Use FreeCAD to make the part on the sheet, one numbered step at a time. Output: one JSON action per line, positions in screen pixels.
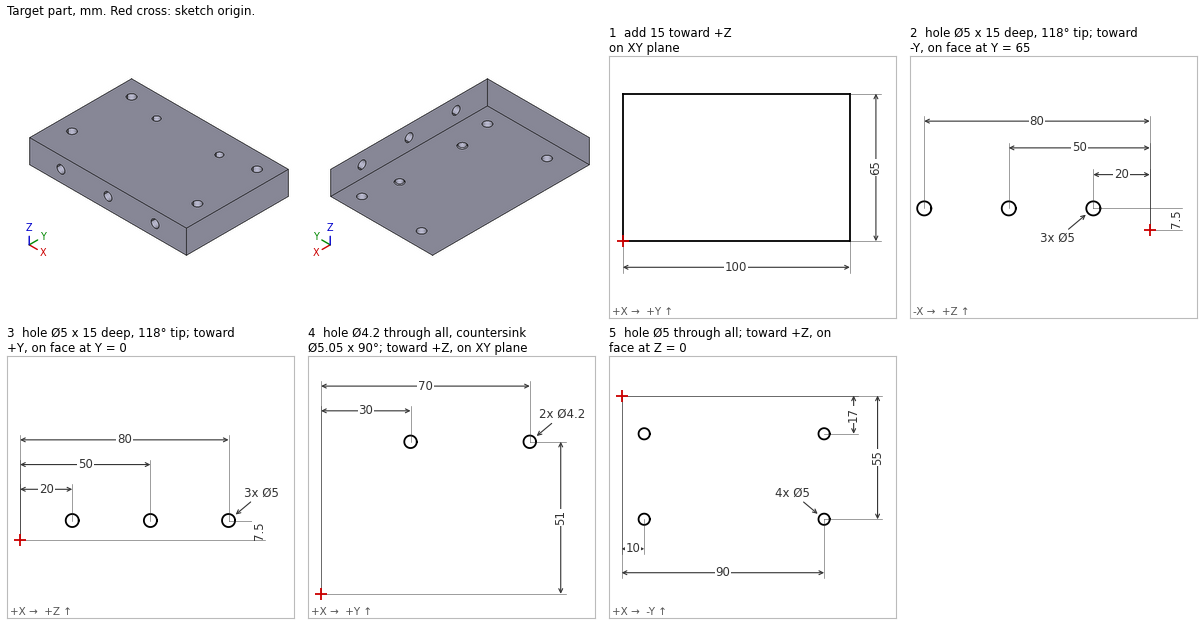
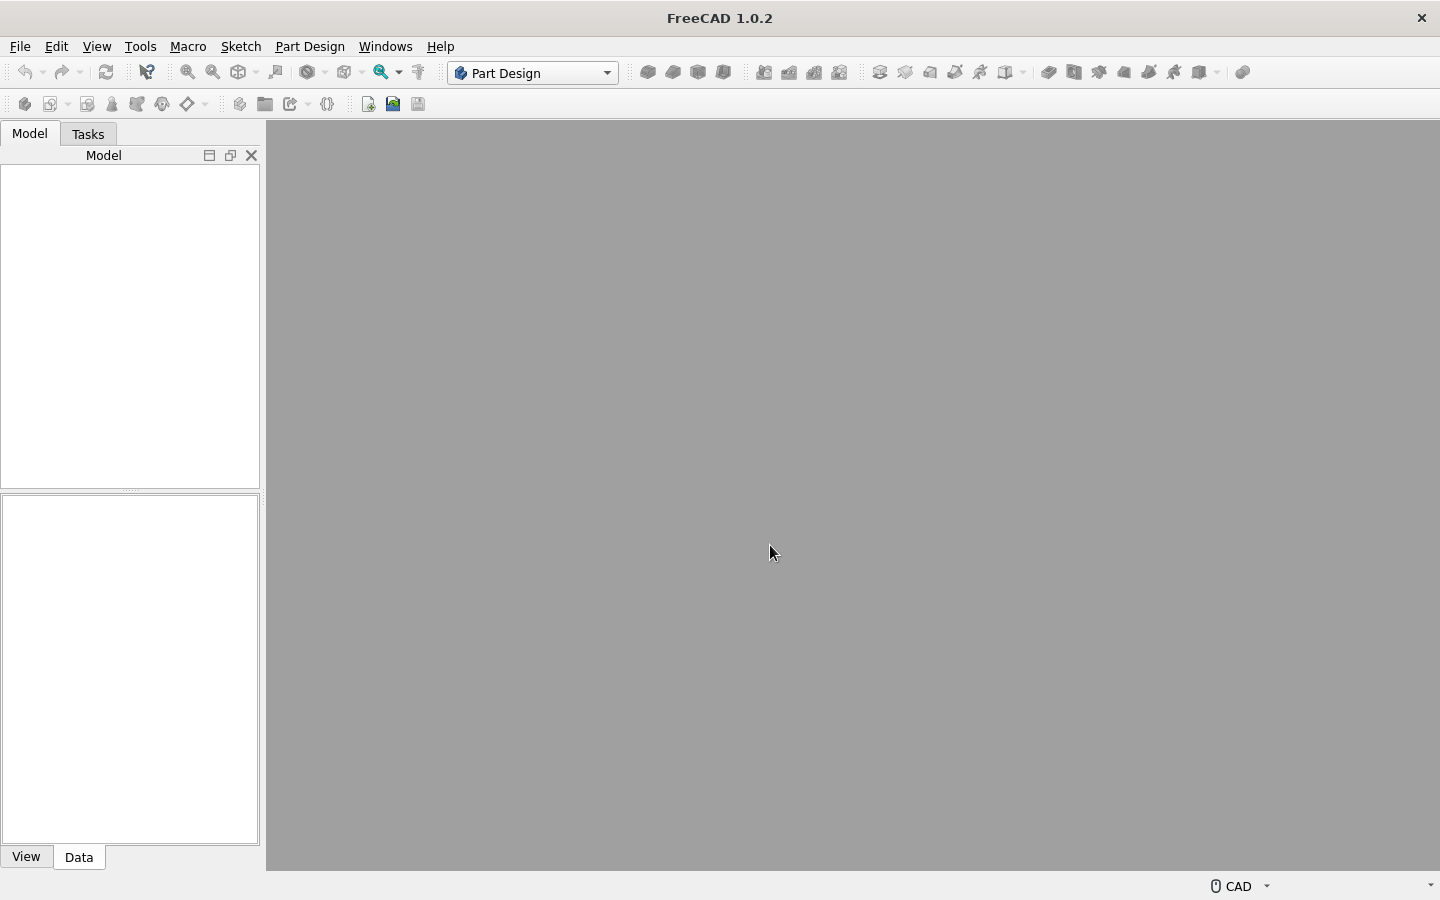
{"action": "left_click", "coordinate": [368, 104]}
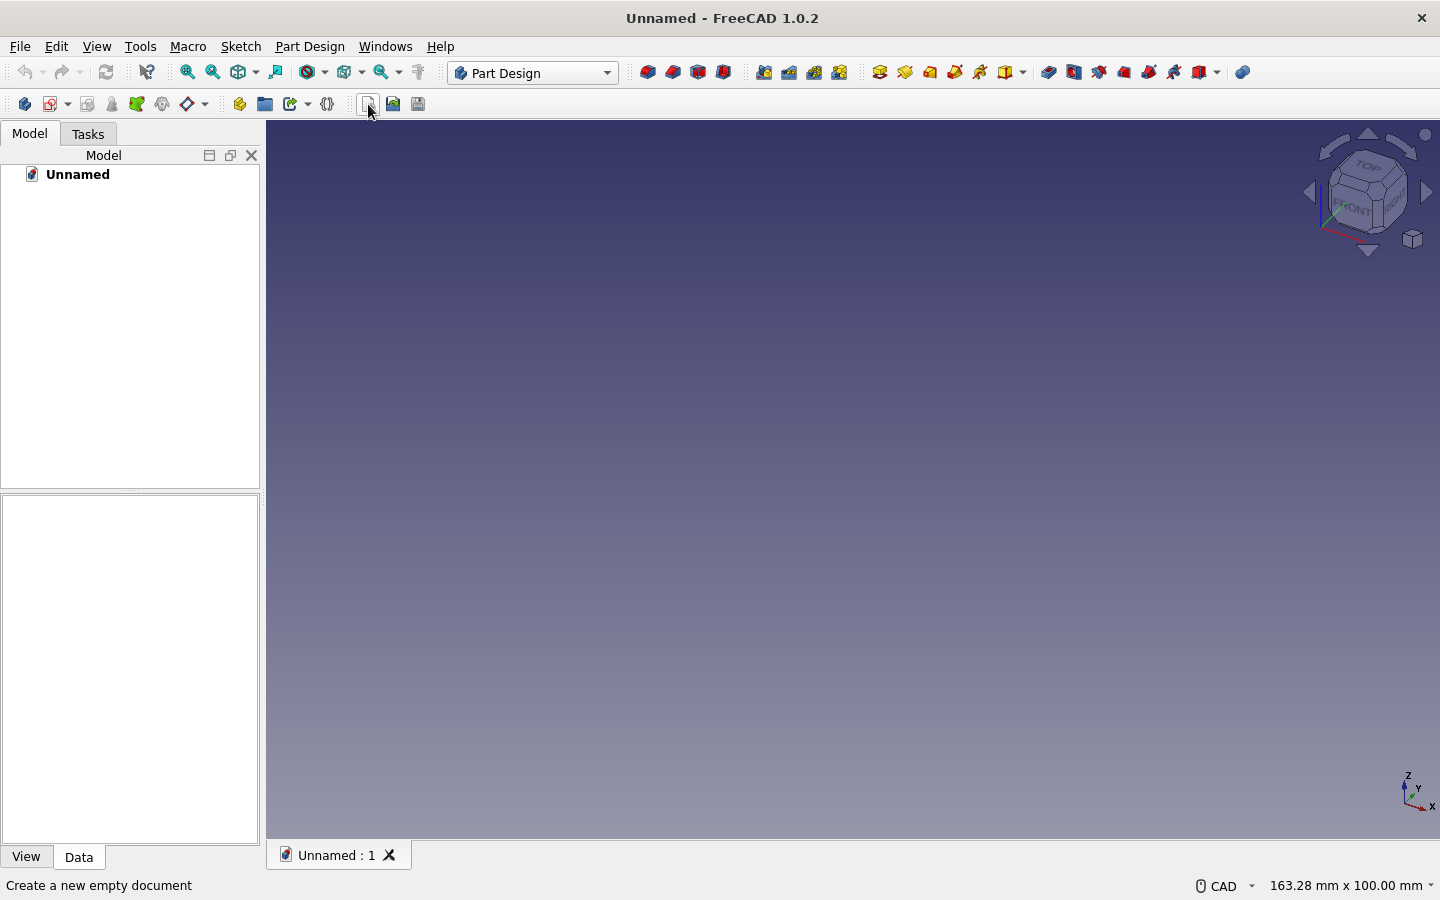
{"action": "left_click", "coordinate": [50, 104]}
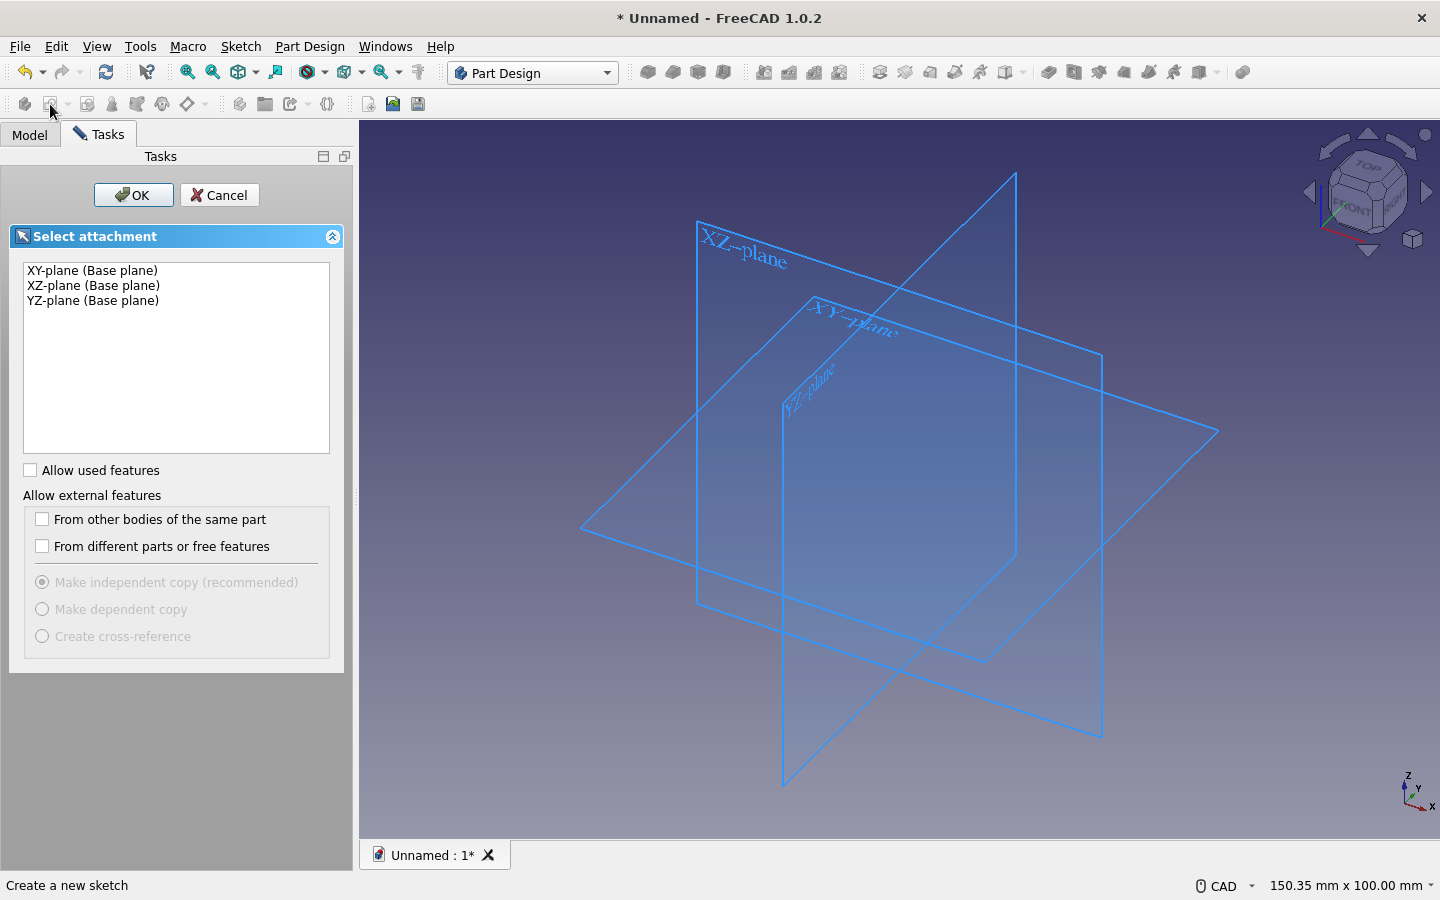
{"action": "left_click", "coordinate": [84, 270]}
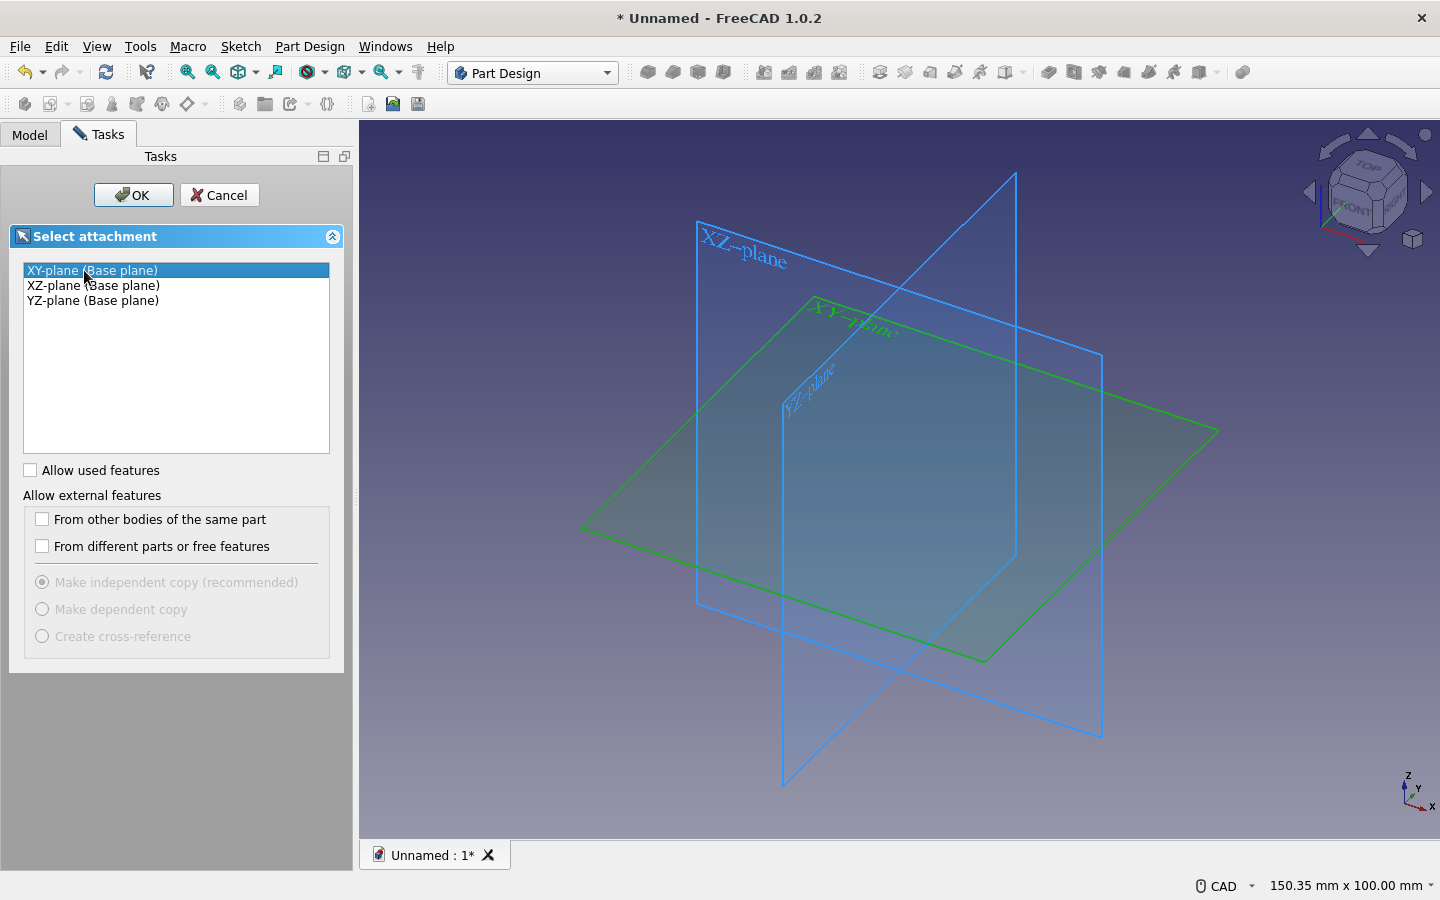
{"action": "left_click", "coordinate": [134, 195]}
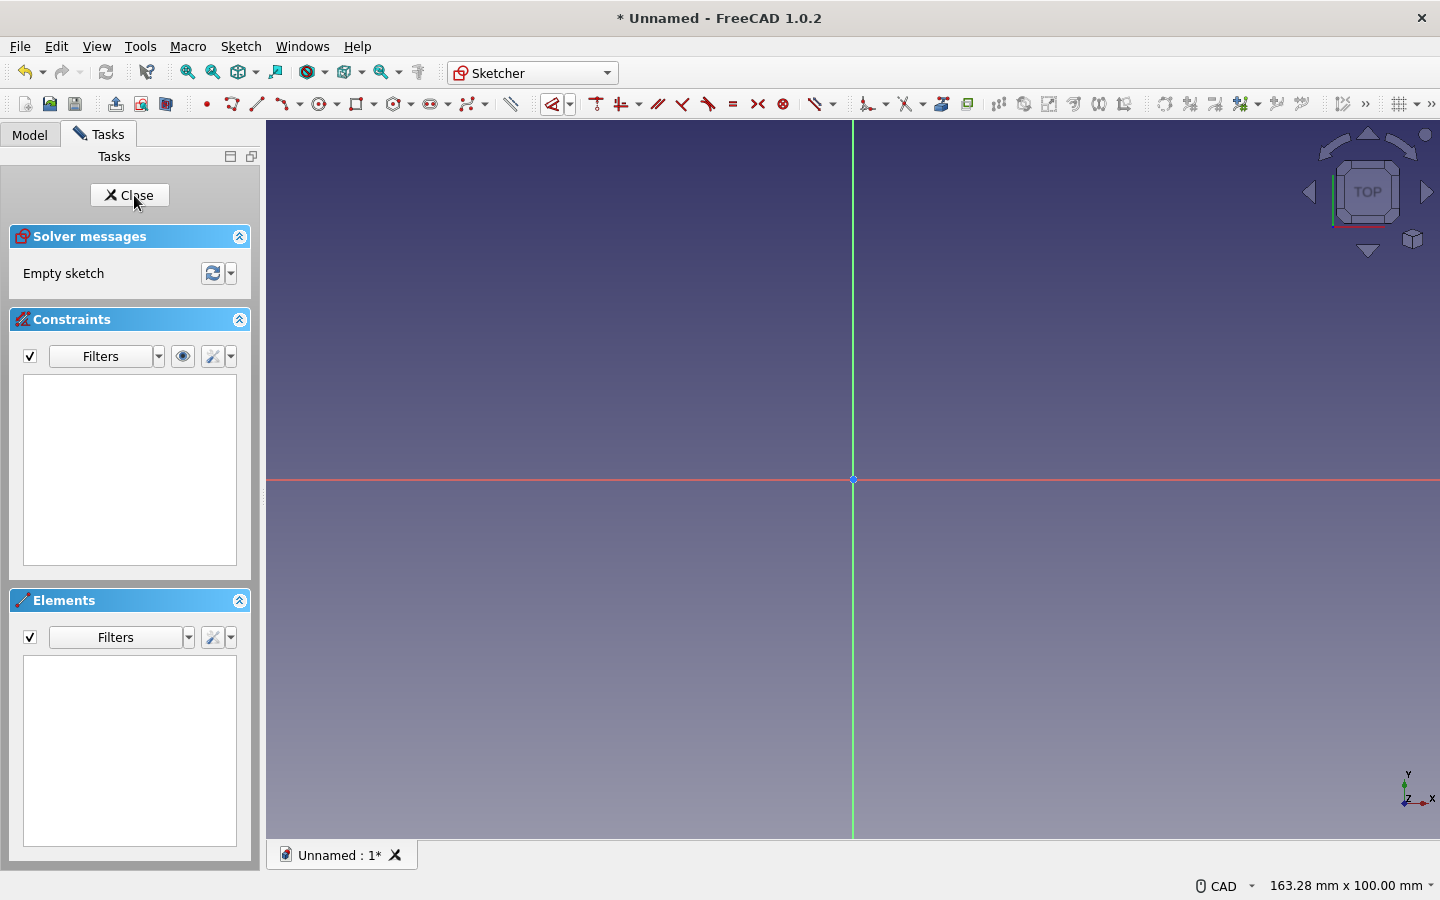
{"action": "scroll", "coordinate": [294, 811], "scroll_direction": "down", "scroll_amount": 2}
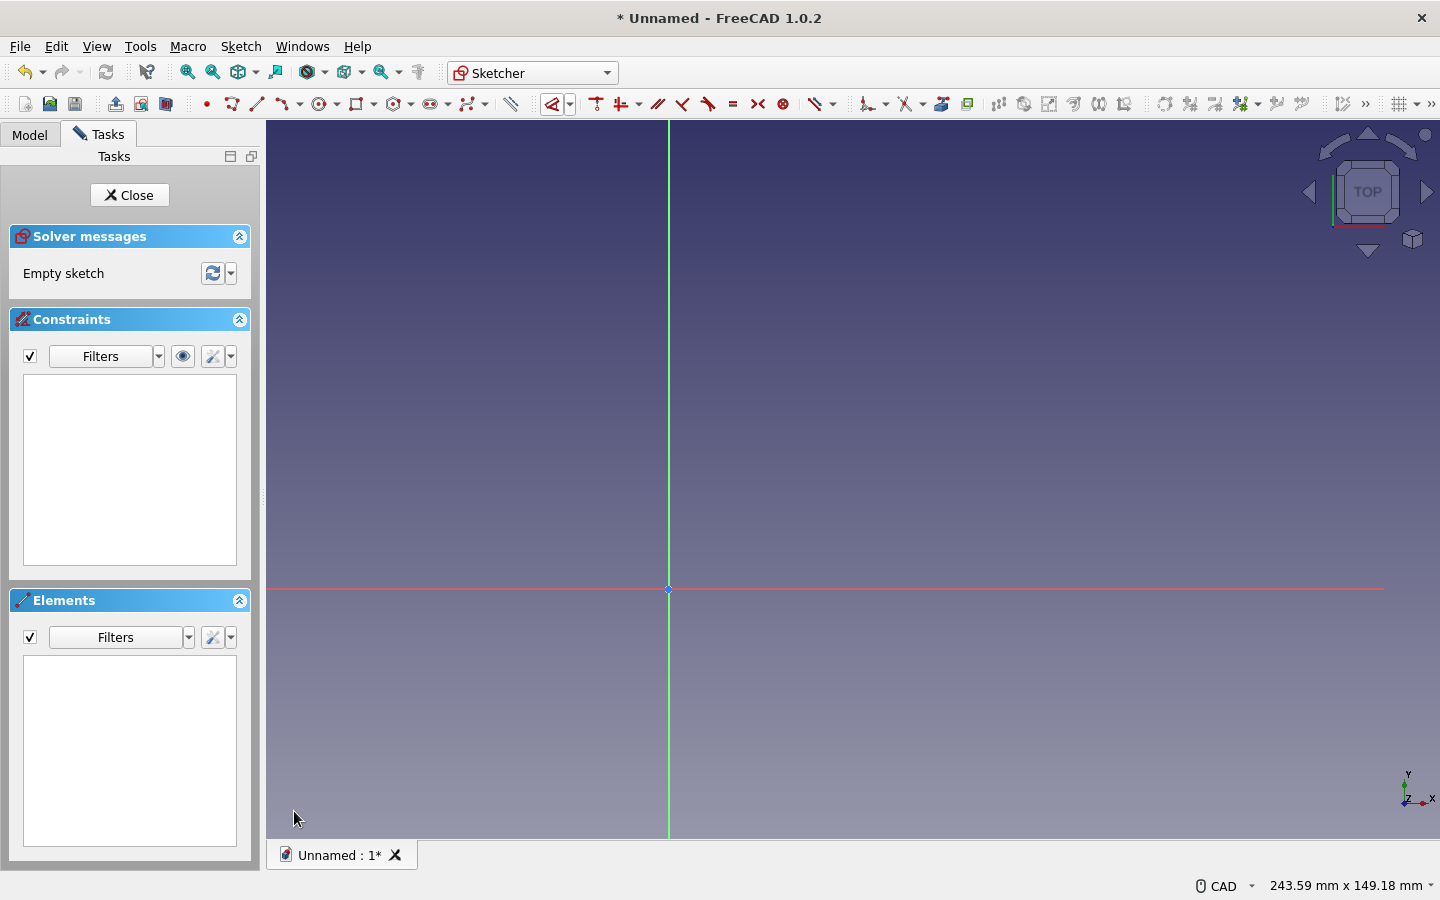
{"action": "scroll", "coordinate": [1164, 337], "scroll_direction": "up", "scroll_amount": 2}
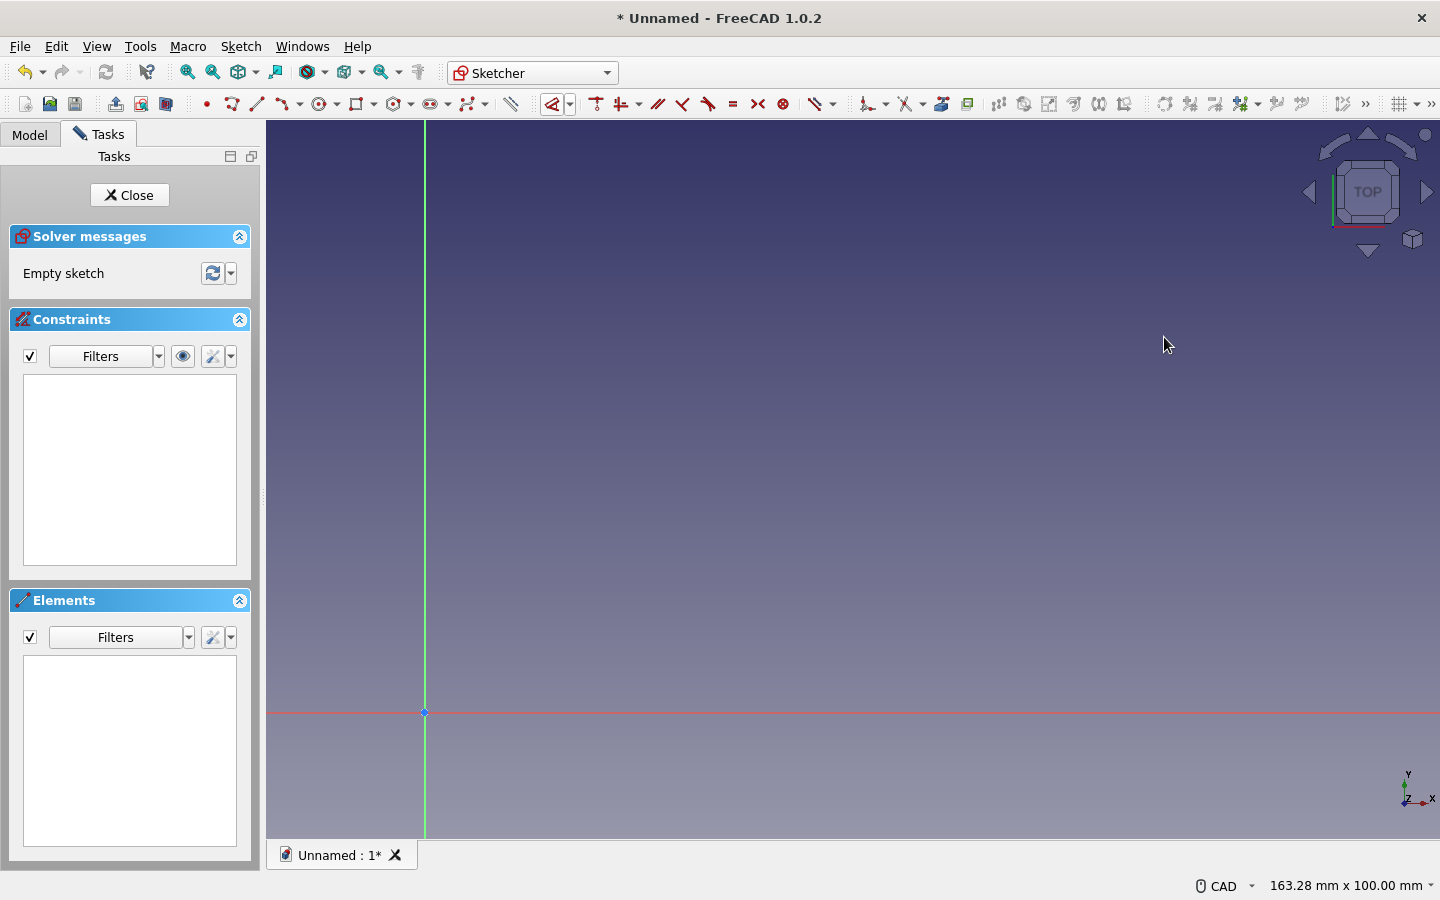
{"action": "left_click", "coordinate": [356, 104]}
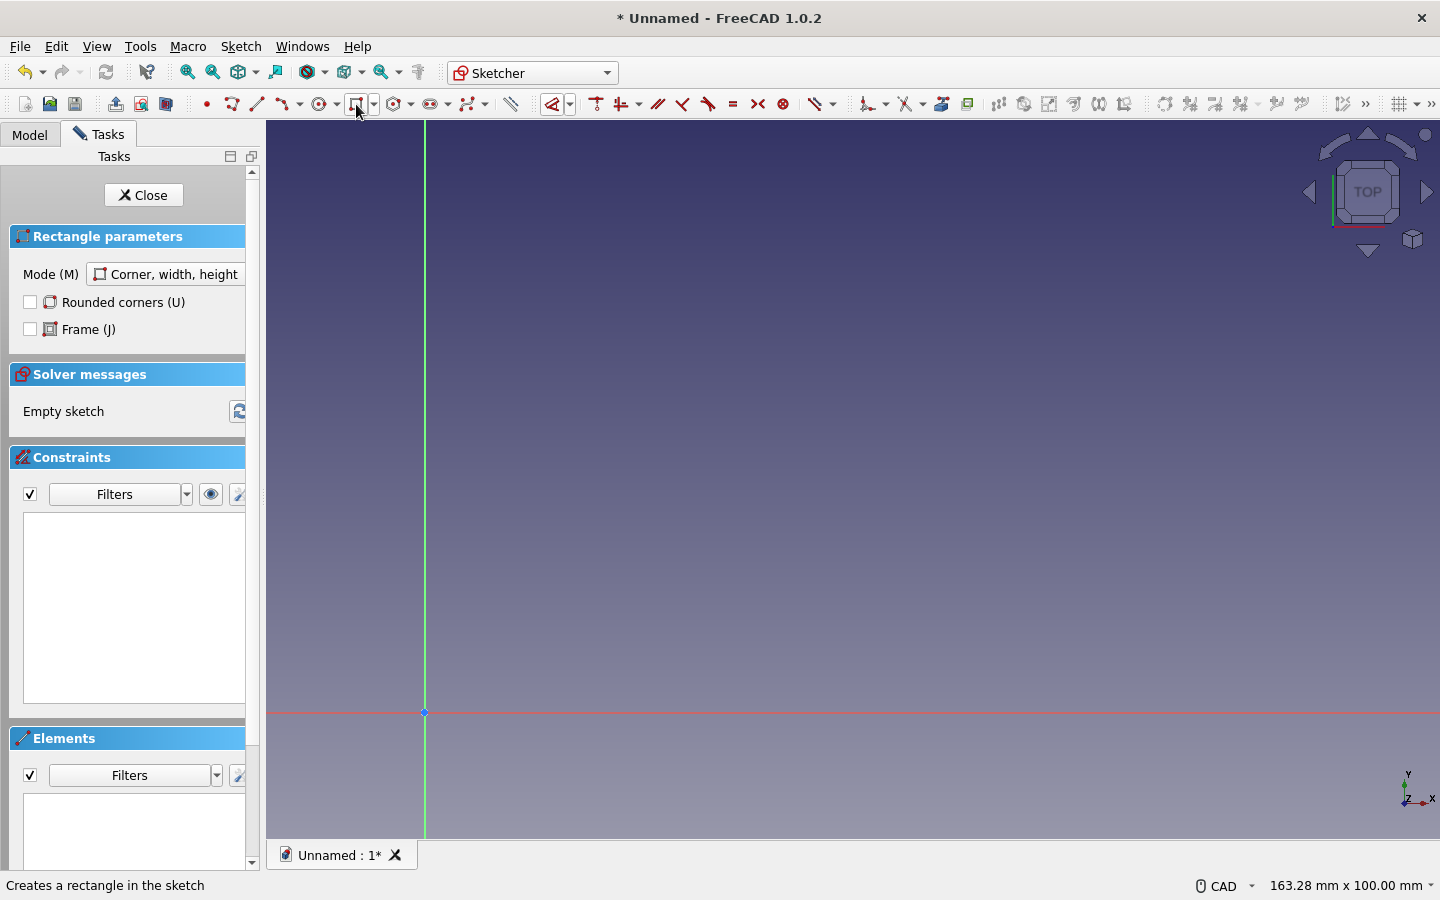
{"action": "left_click", "coordinate": [425, 713]}
{"action": "mouse_move", "coordinate": [1144, 246]}